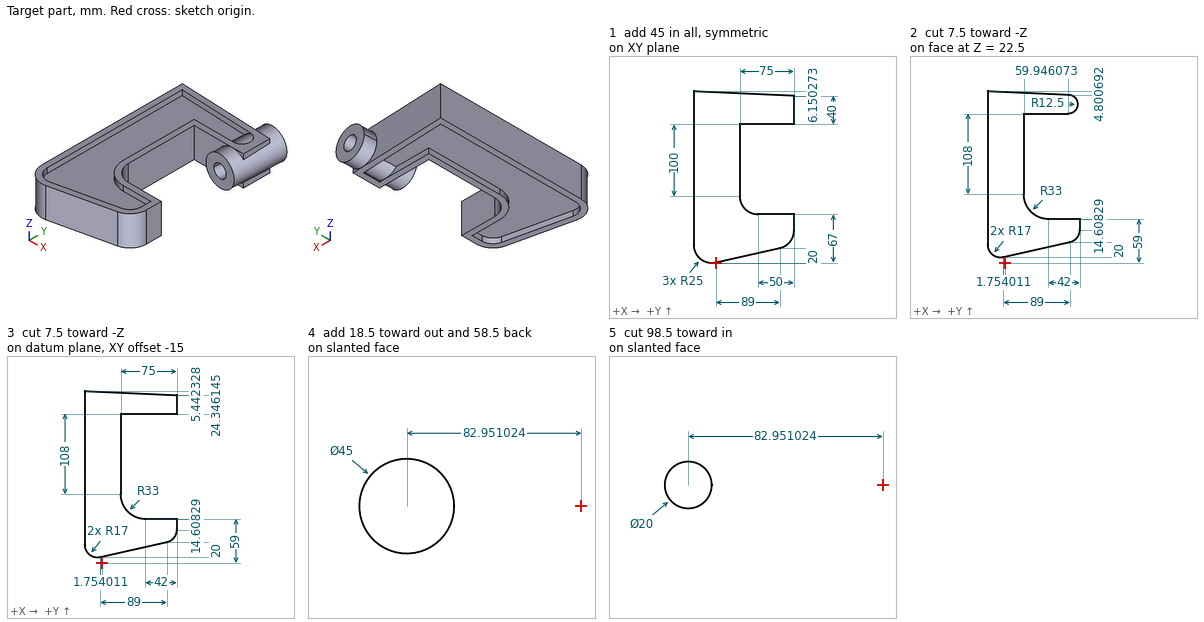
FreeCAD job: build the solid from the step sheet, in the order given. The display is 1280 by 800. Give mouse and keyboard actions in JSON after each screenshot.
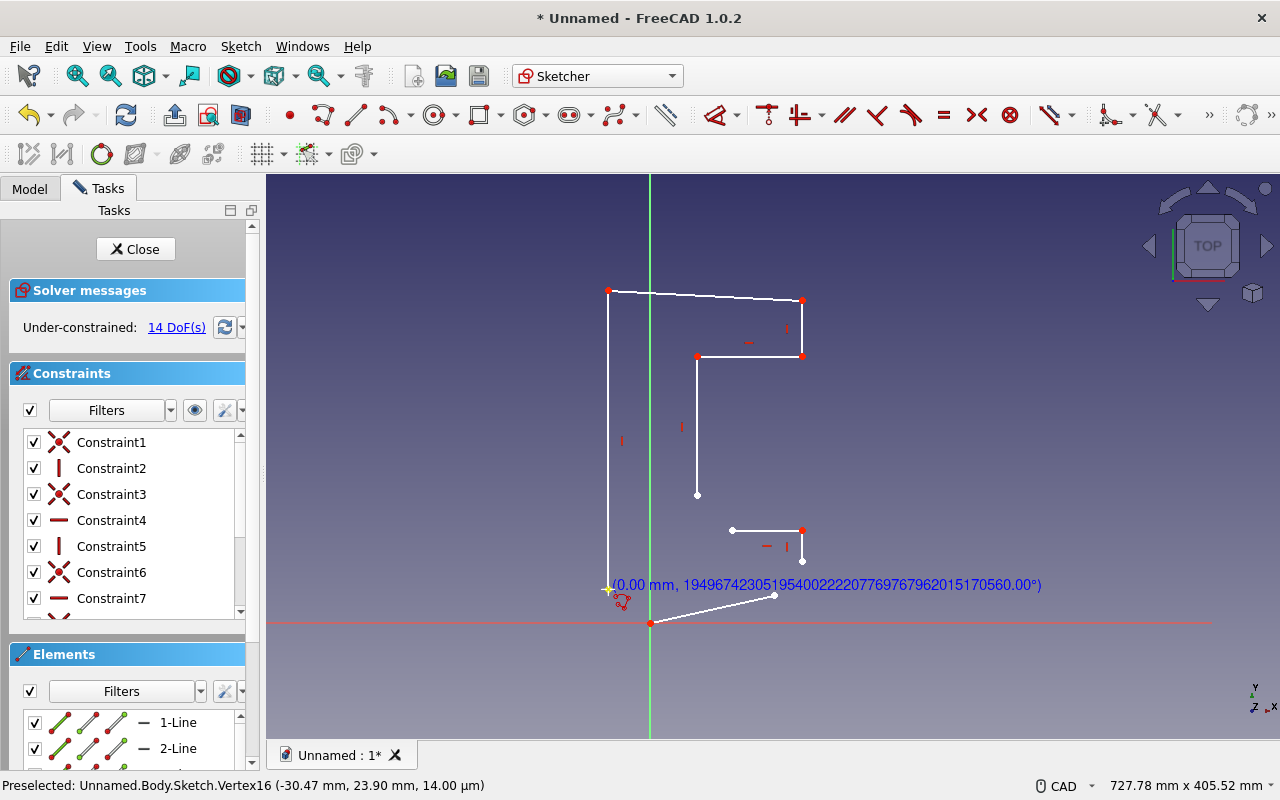
{"action": "key", "text": "g 3 a"}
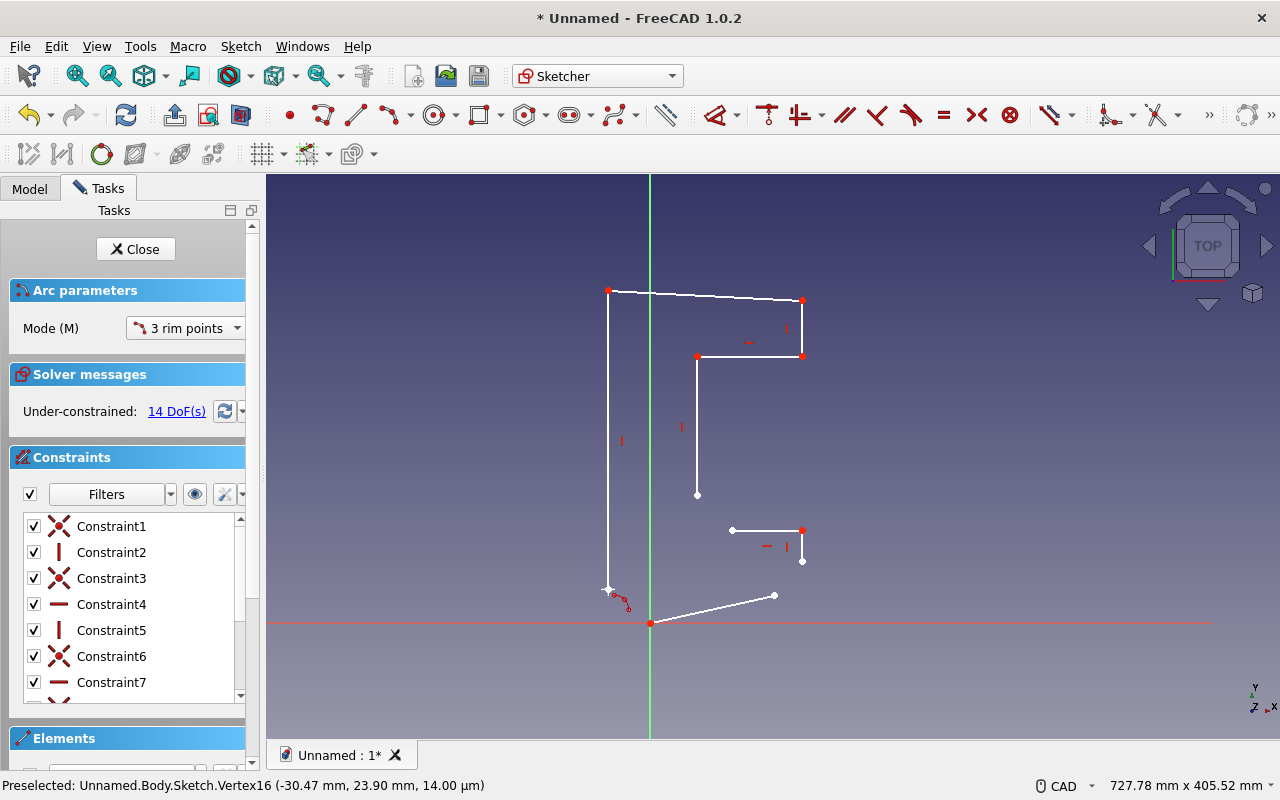
{"action": "left_click", "coordinate": [774, 596]}
{"action": "left_click", "coordinate": [802, 562]}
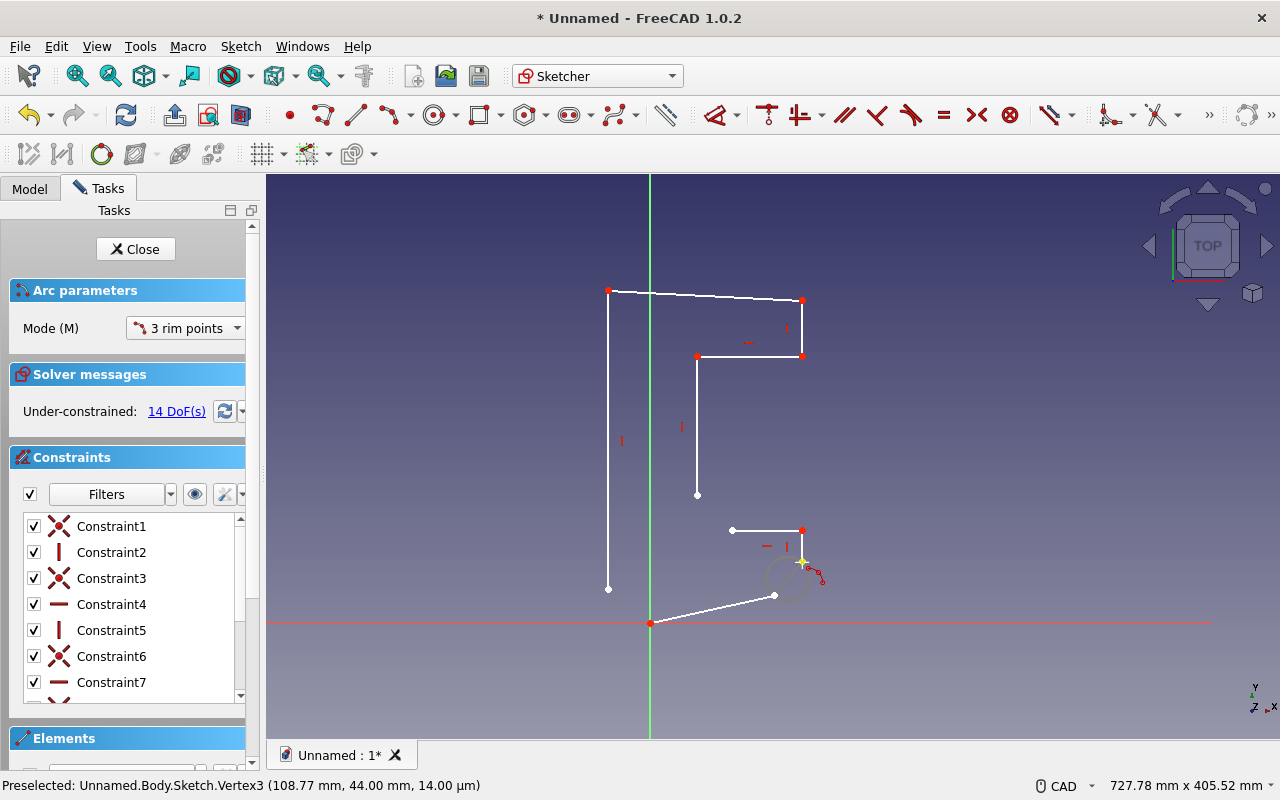
{"action": "scroll", "coordinate": [794, 583], "scroll_direction": "up", "scroll_amount": 4}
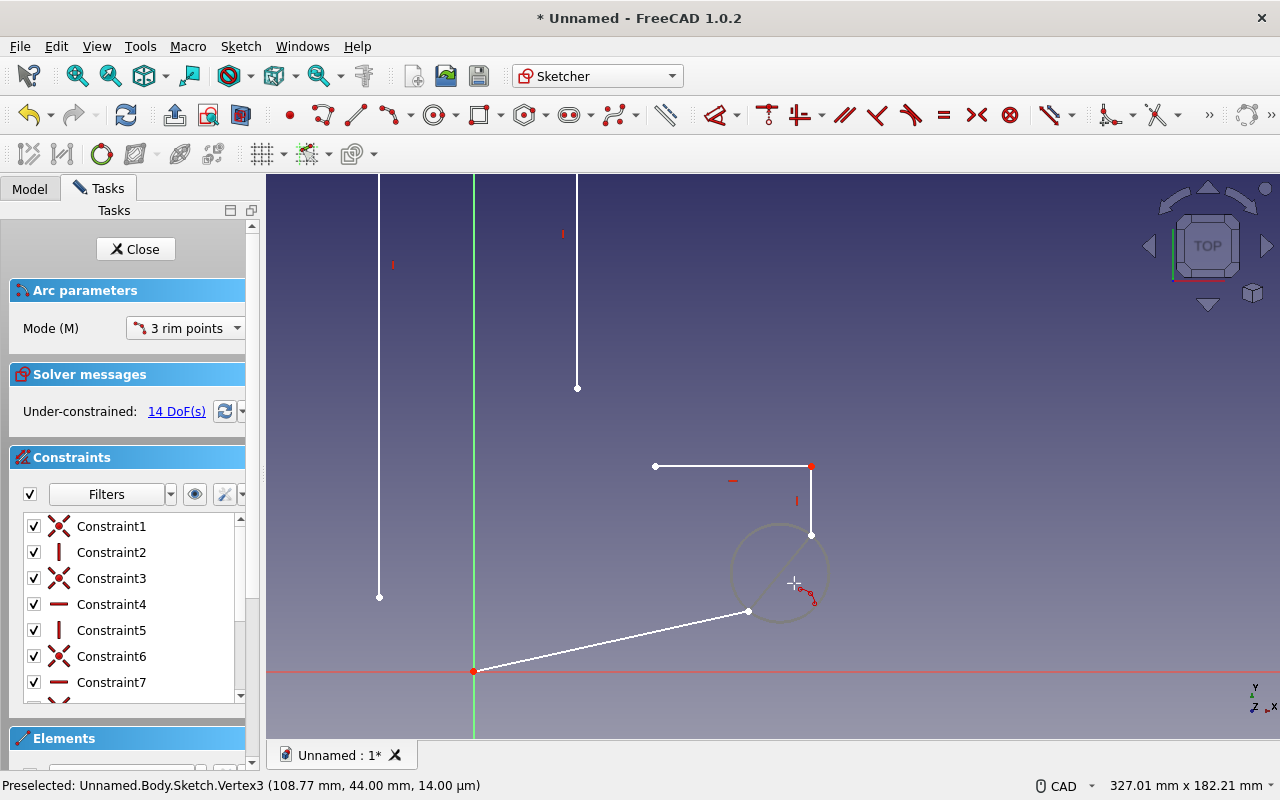
{"action": "left_click", "coordinate": [793, 583]}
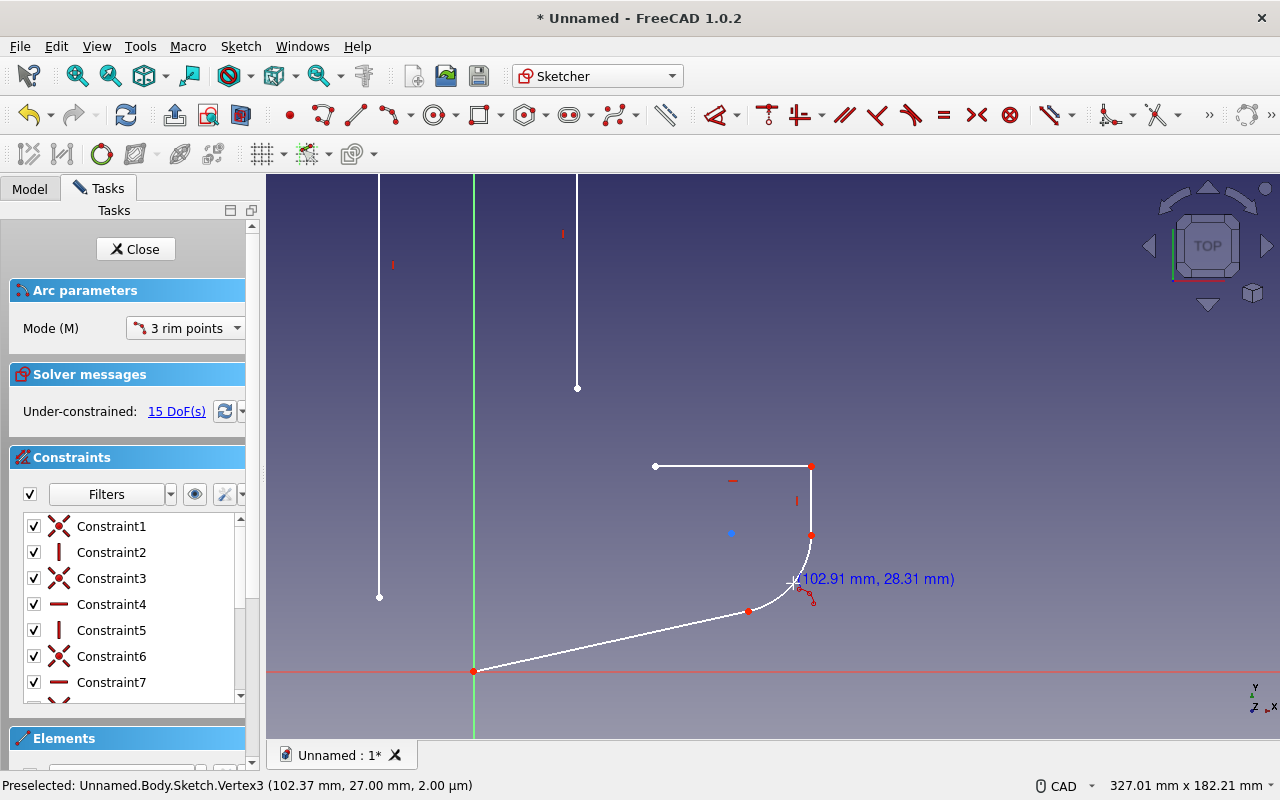
{"action": "left_click", "coordinate": [655, 466]}
{"action": "left_click", "coordinate": [577, 388]}
{"action": "left_click", "coordinate": [601, 441]}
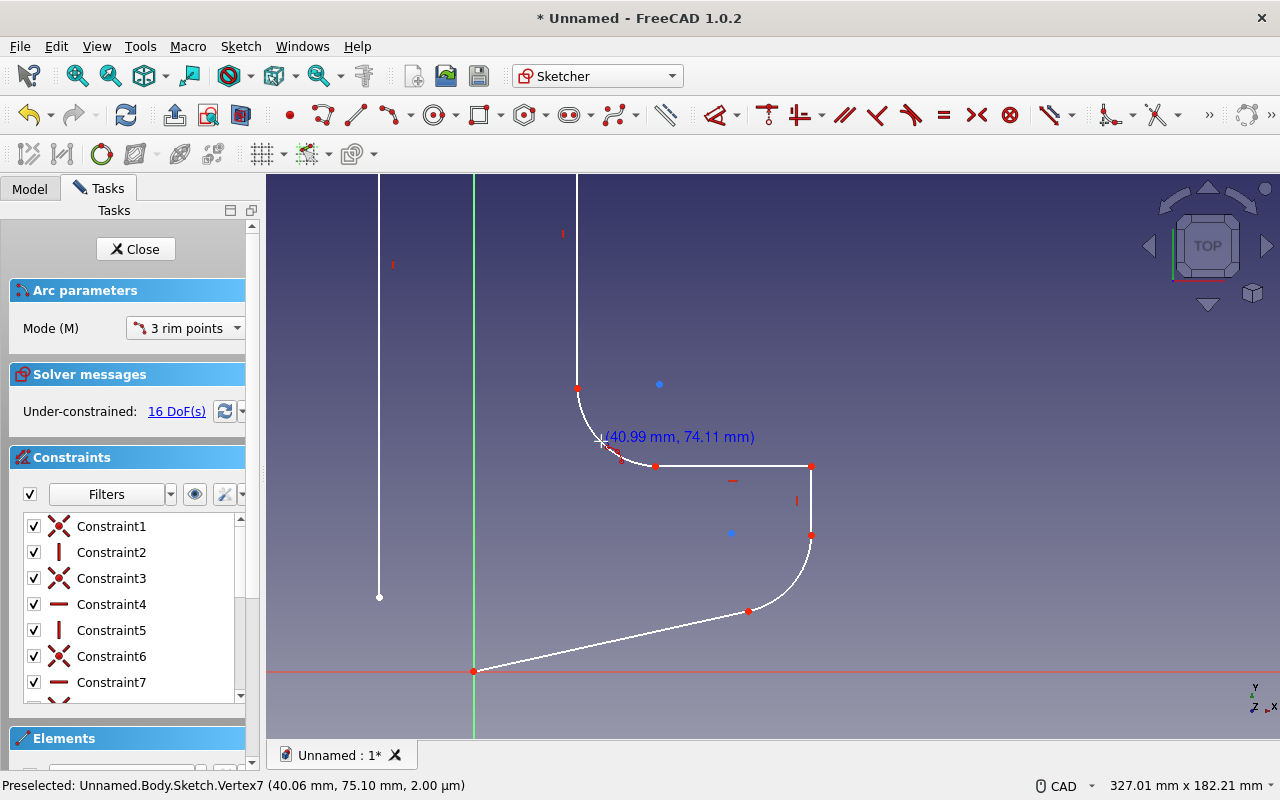
{"action": "left_click", "coordinate": [379, 598]}
{"action": "left_click", "coordinate": [474, 672]}
{"action": "left_click", "coordinate": [398, 647]}
{"action": "key", "text": "Escape"}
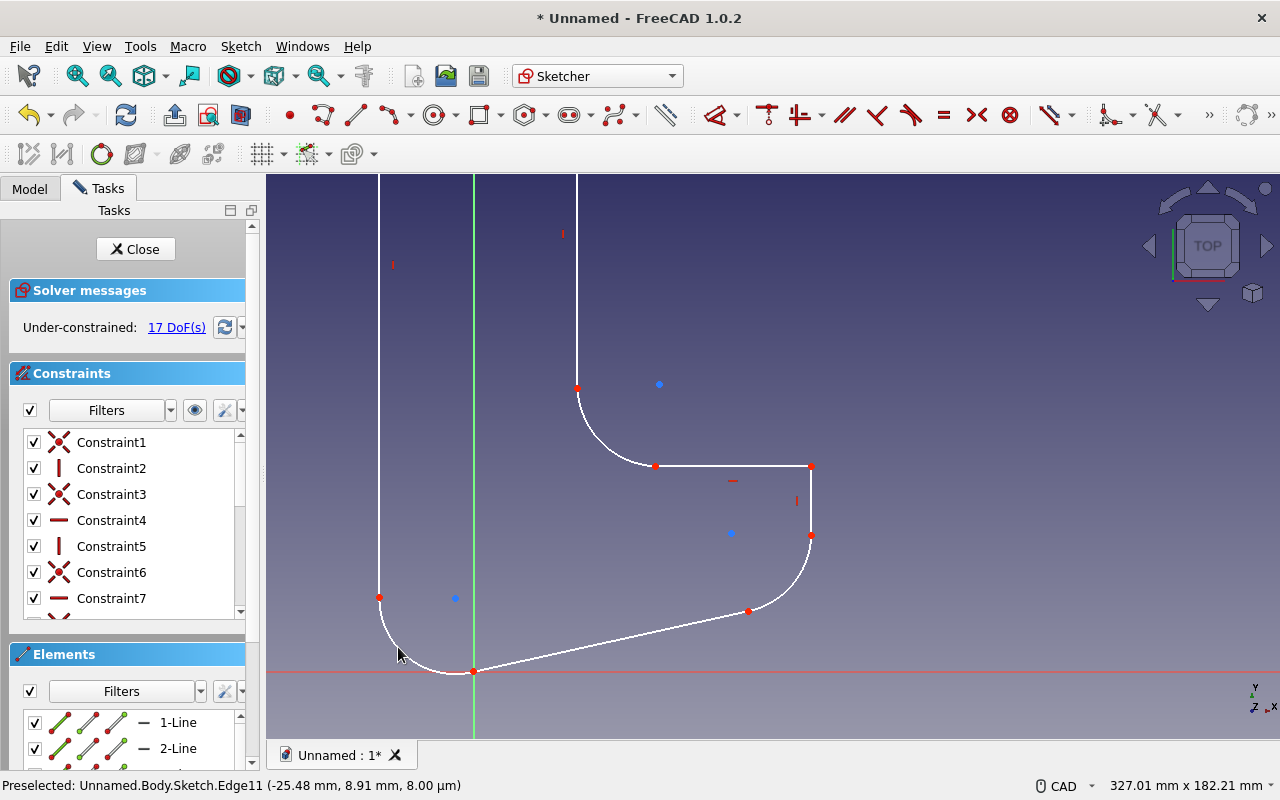
{"action": "left_click", "coordinate": [556, 654]}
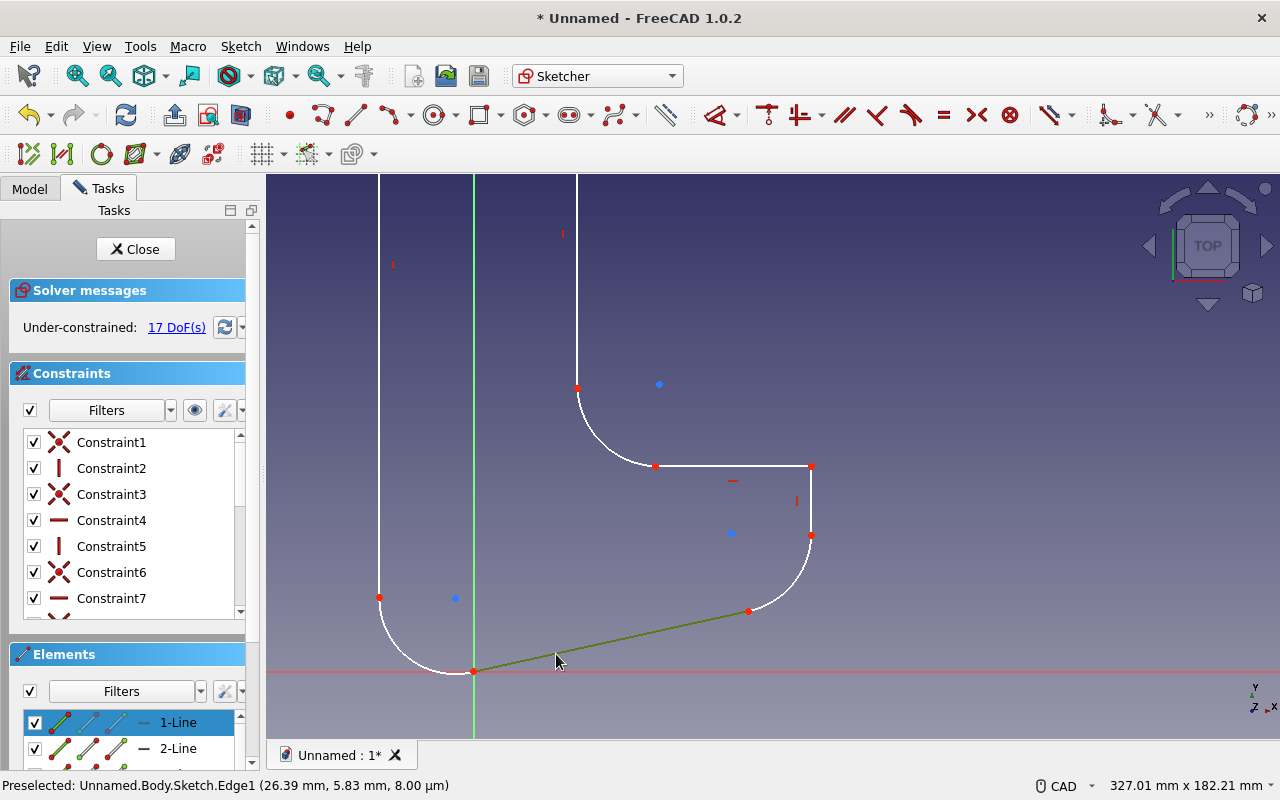
{"action": "left_click", "coordinate": [778, 598]}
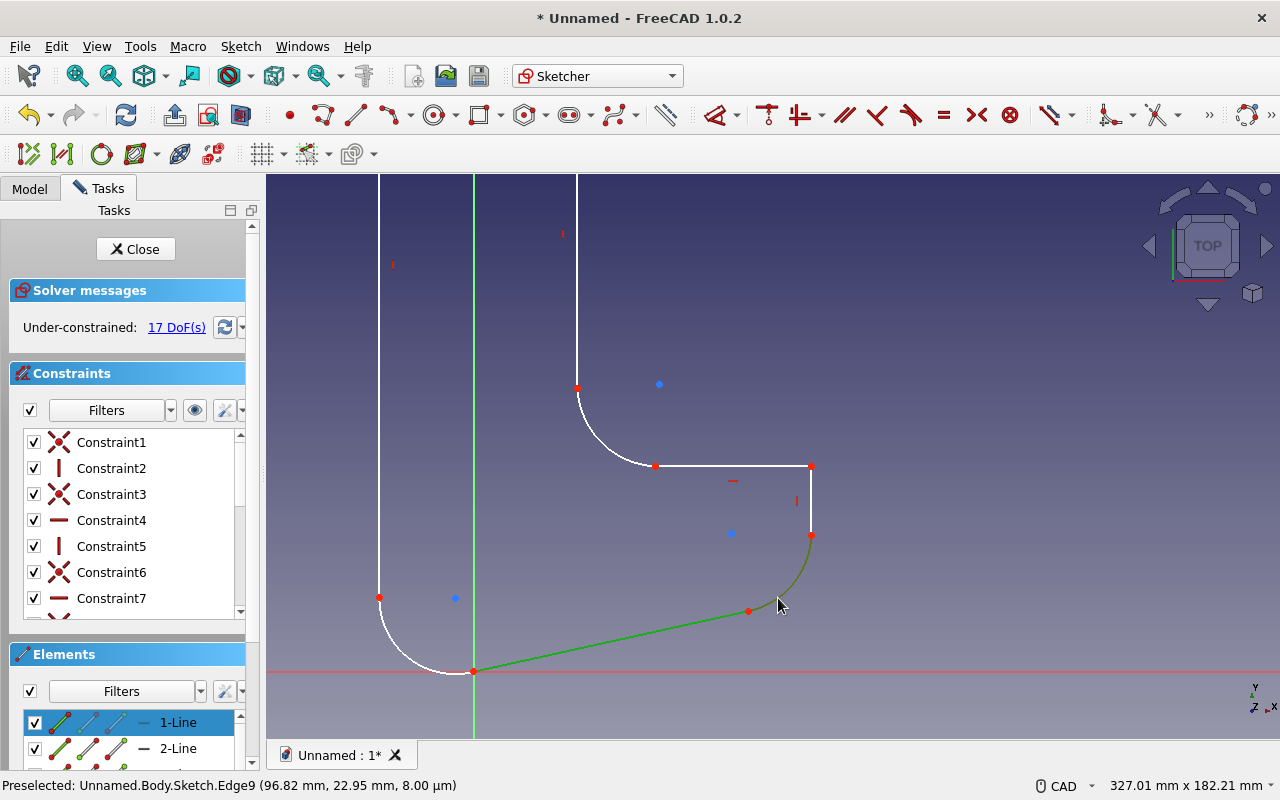
{"action": "left_click", "coordinate": [911, 116]}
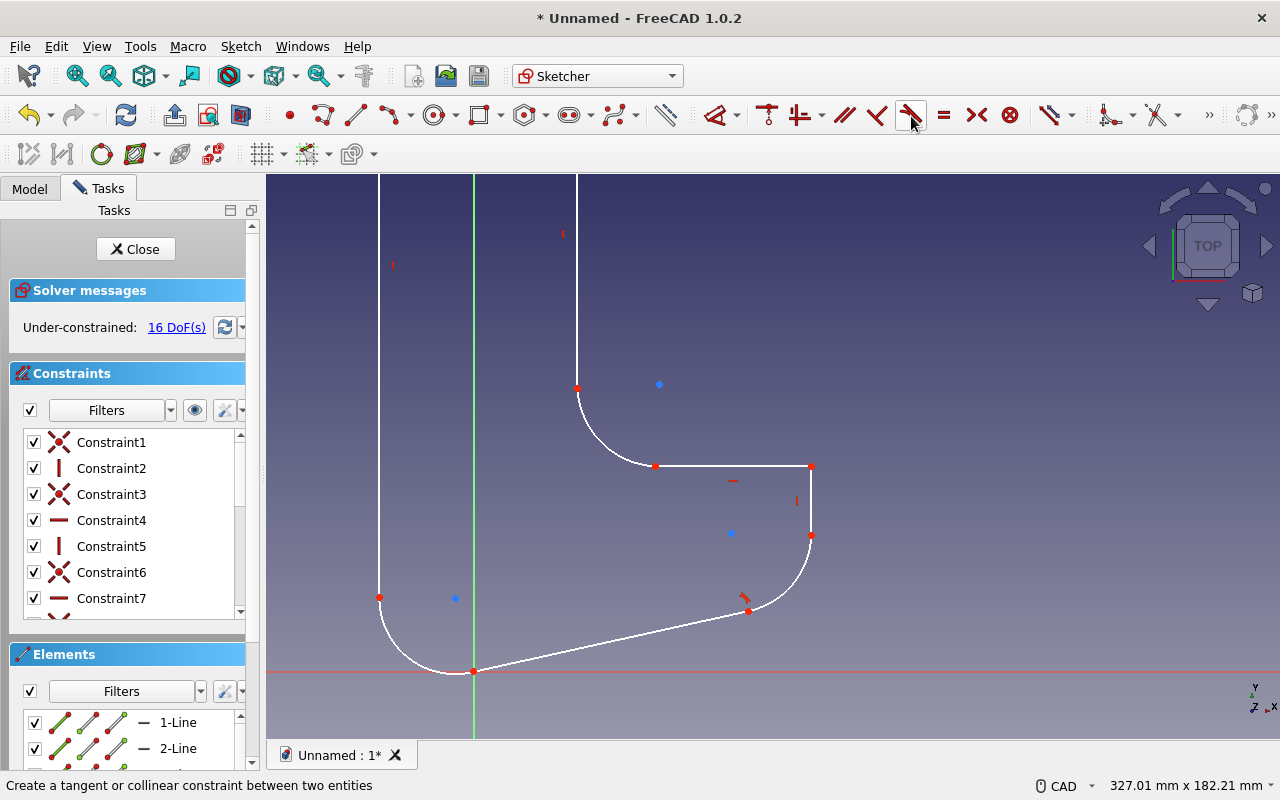
{"action": "left_click", "coordinate": [556, 654]}